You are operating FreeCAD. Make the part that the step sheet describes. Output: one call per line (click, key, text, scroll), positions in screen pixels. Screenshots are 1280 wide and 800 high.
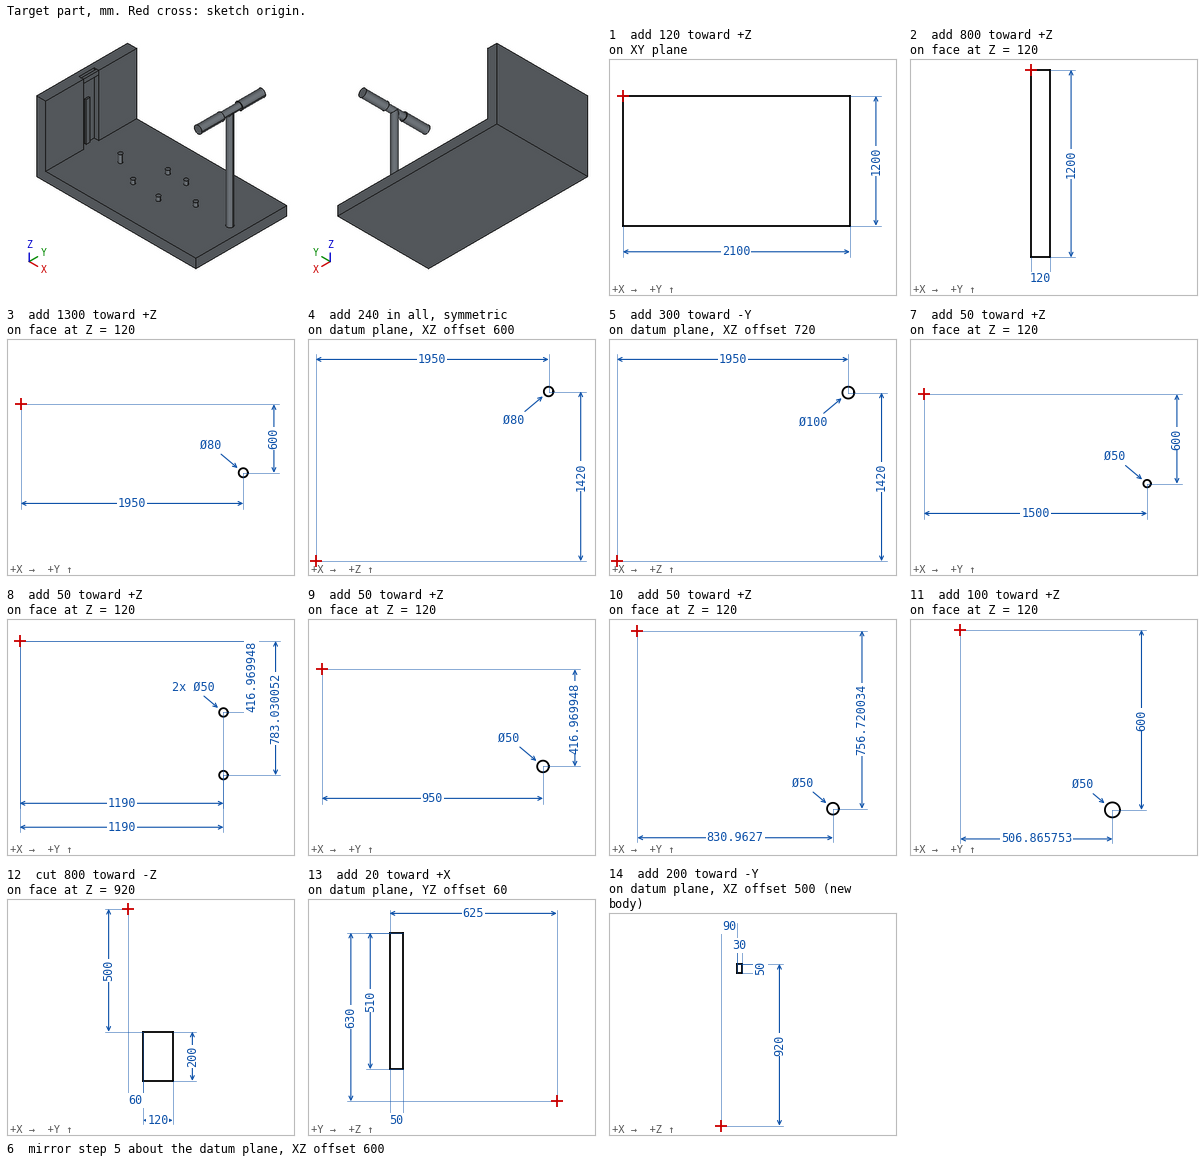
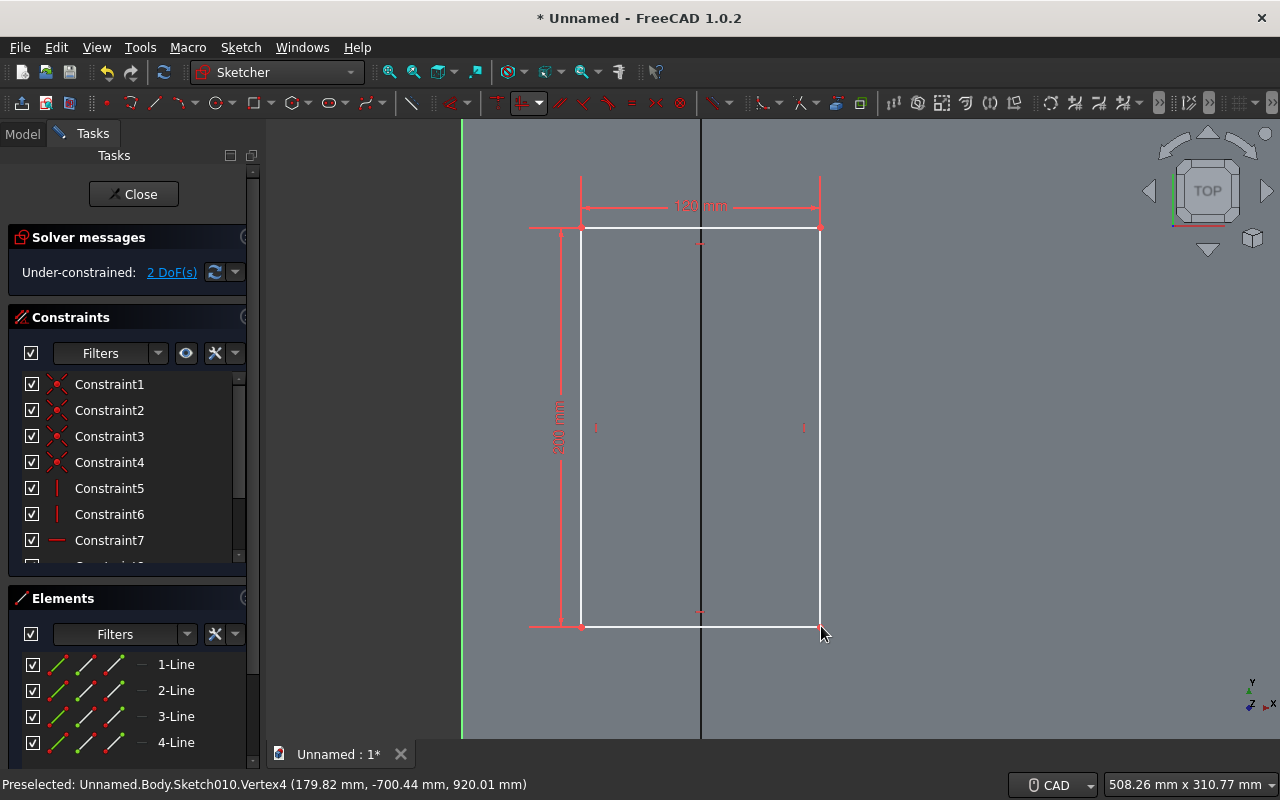
click(450, 104)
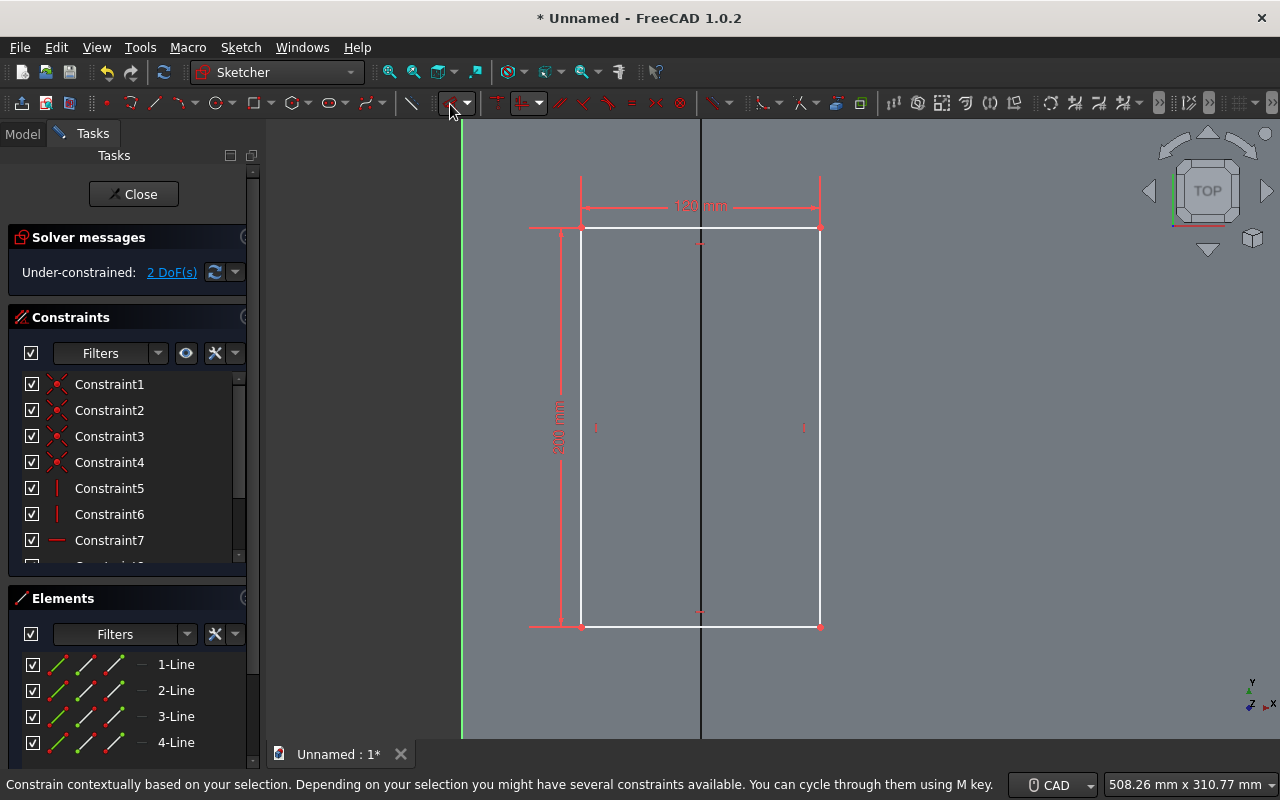
click(581, 228)
click(521, 262)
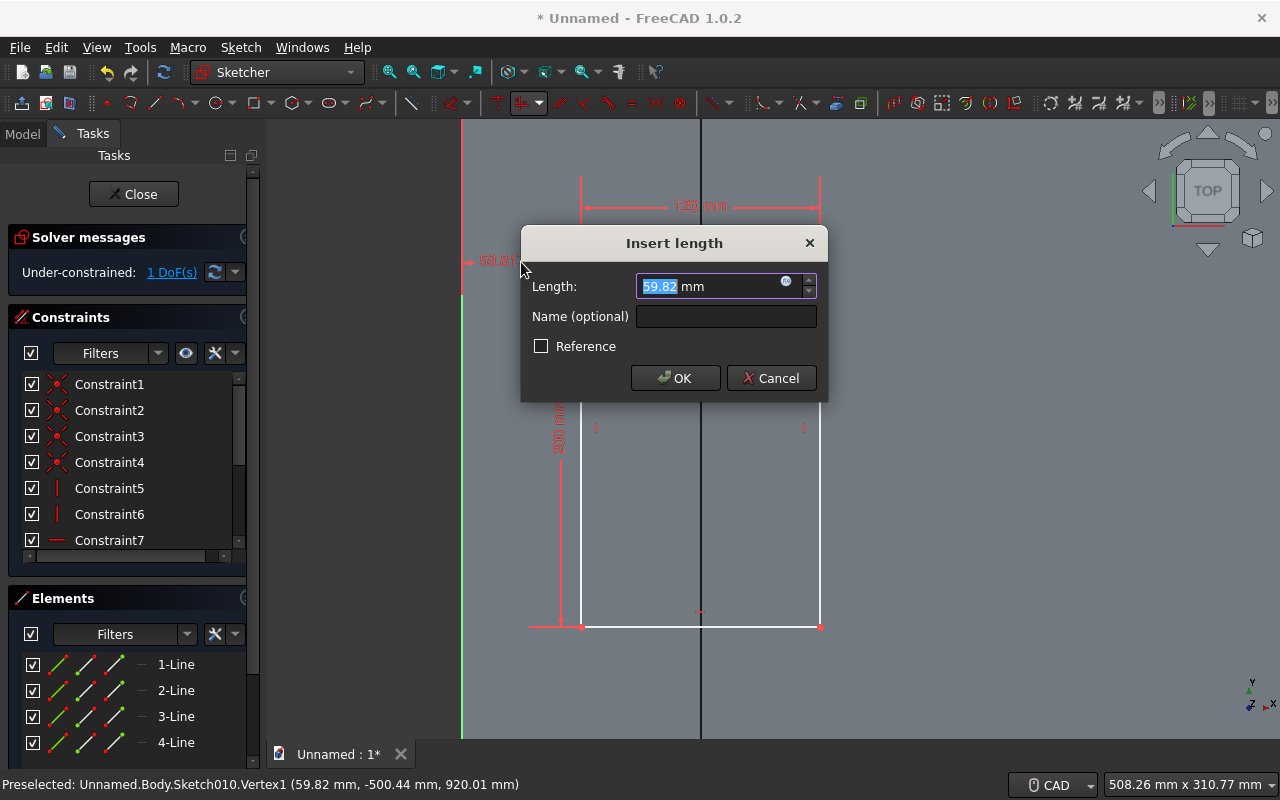
text(60)
key(Return)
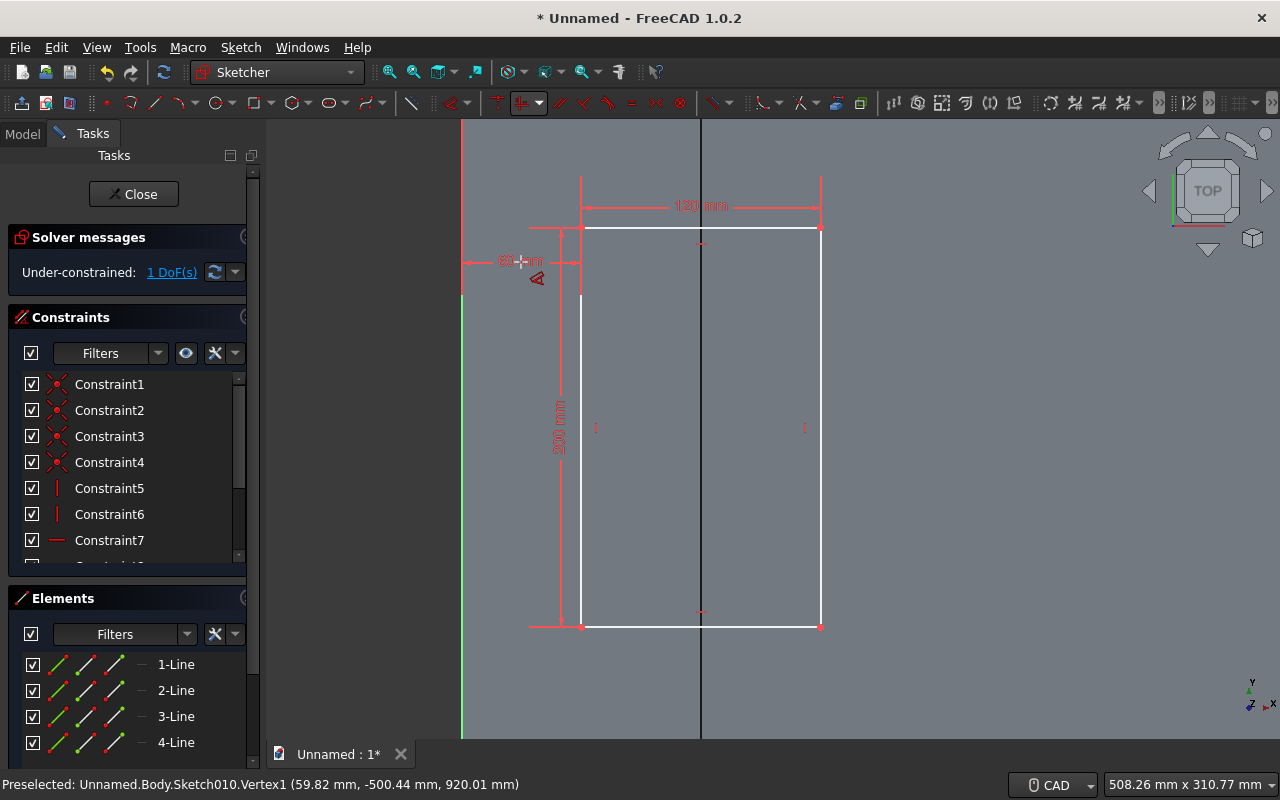
click(581, 228)
click(428, 188)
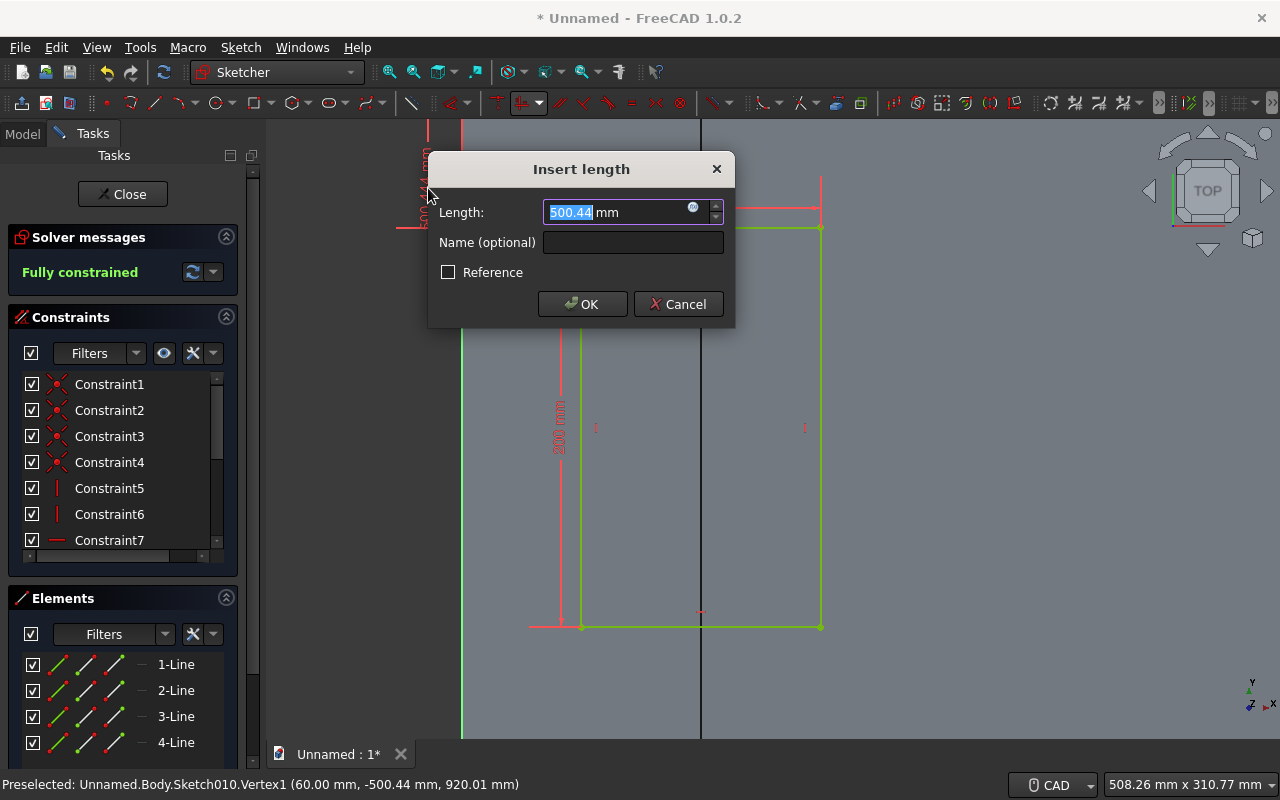
text(500)
key(Return)
key(Escape)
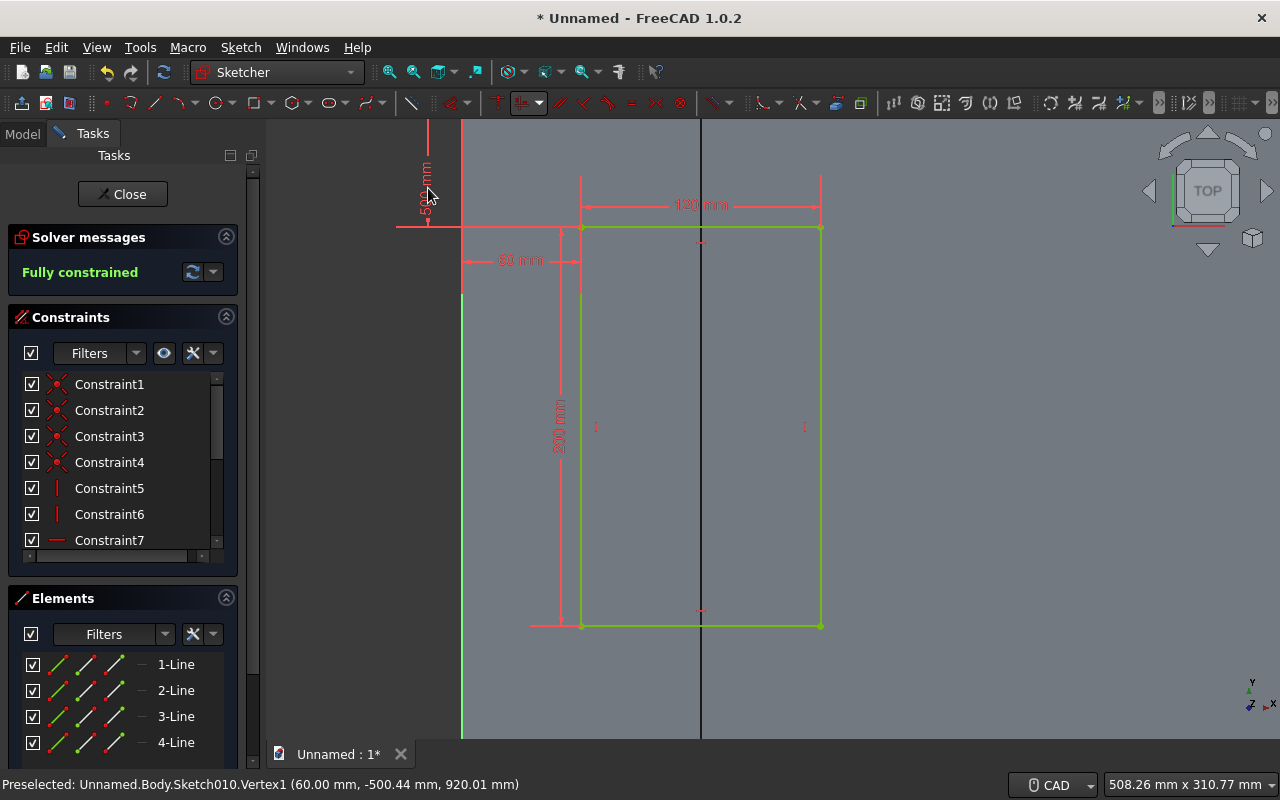
click(123, 194)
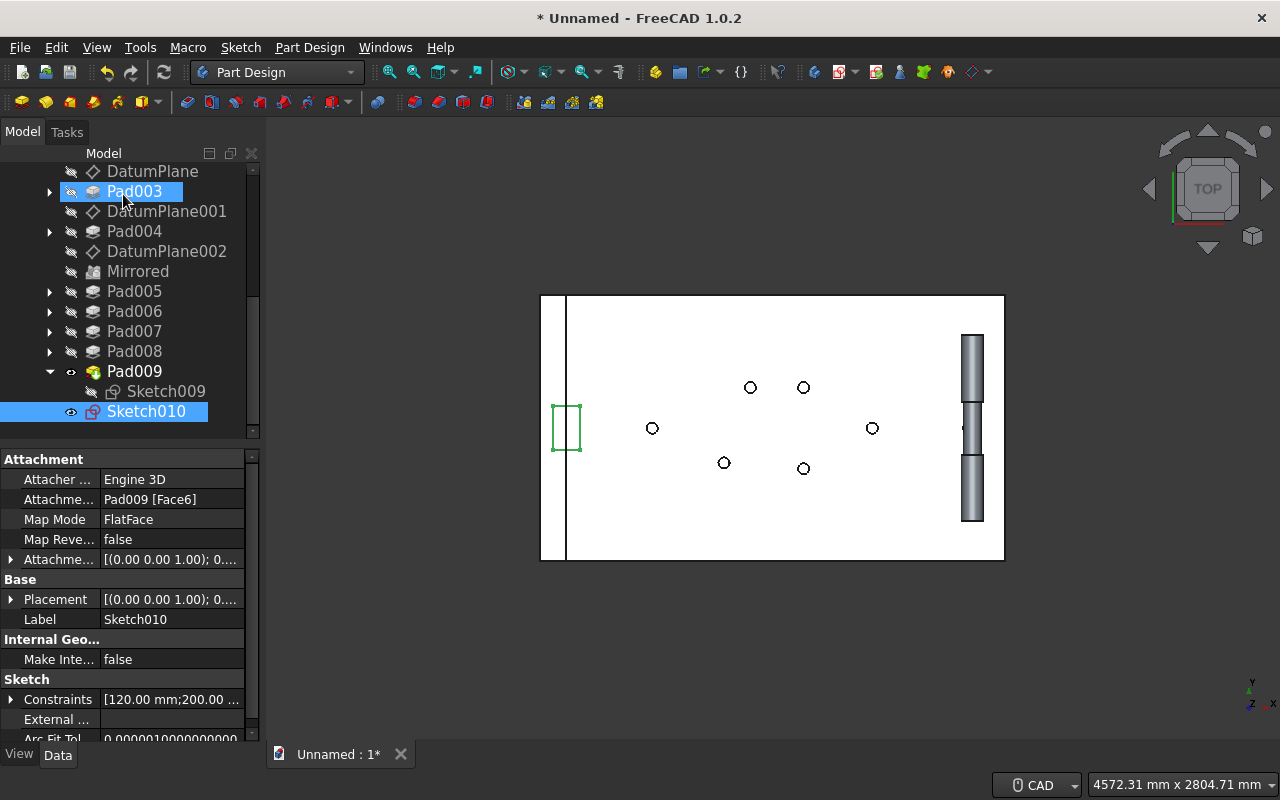
click(188, 102)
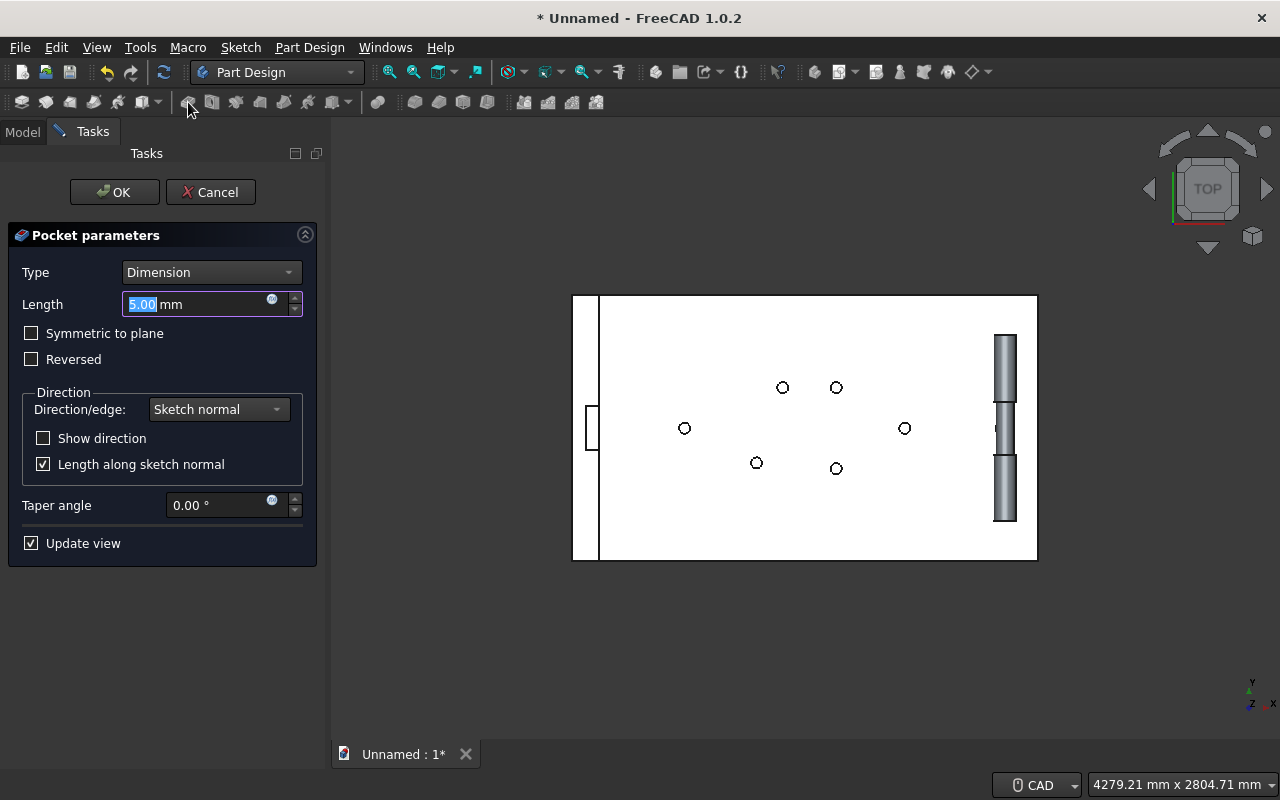
text(800)
key(Tab)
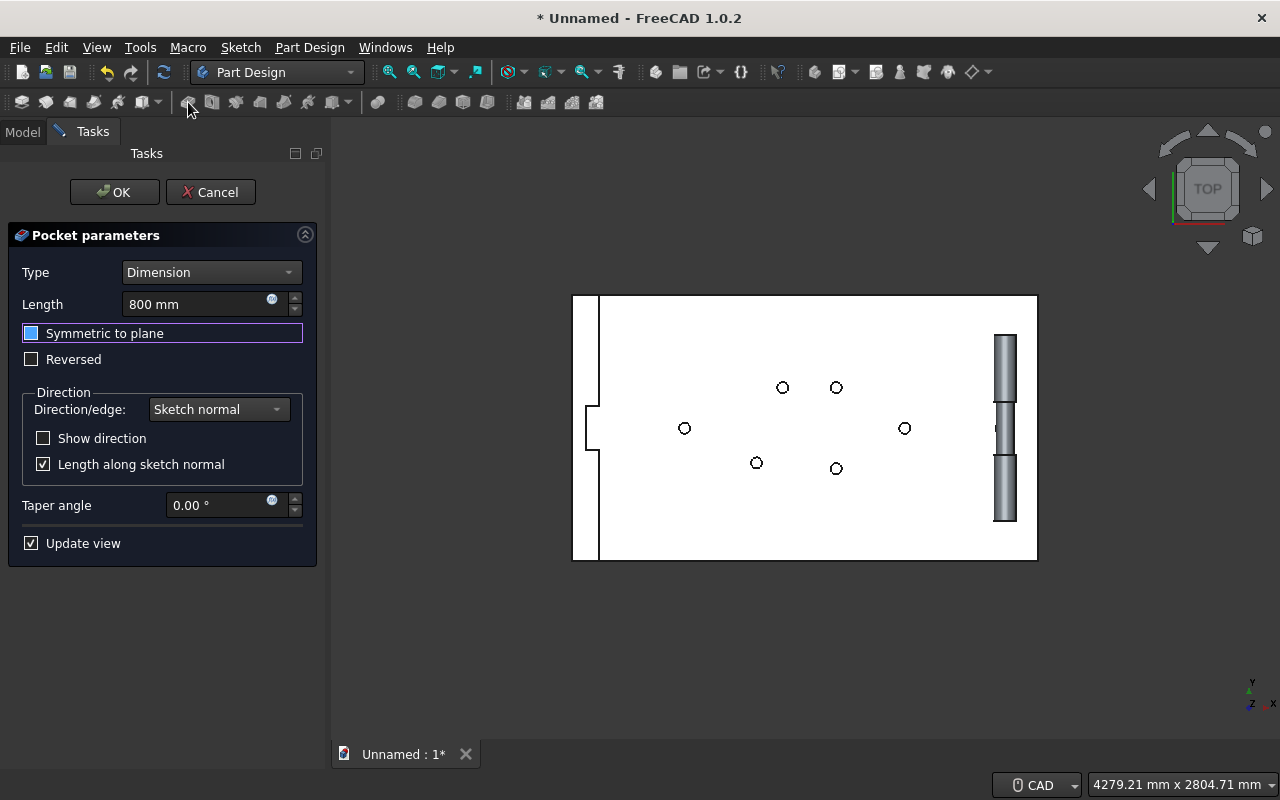
click(115, 192)